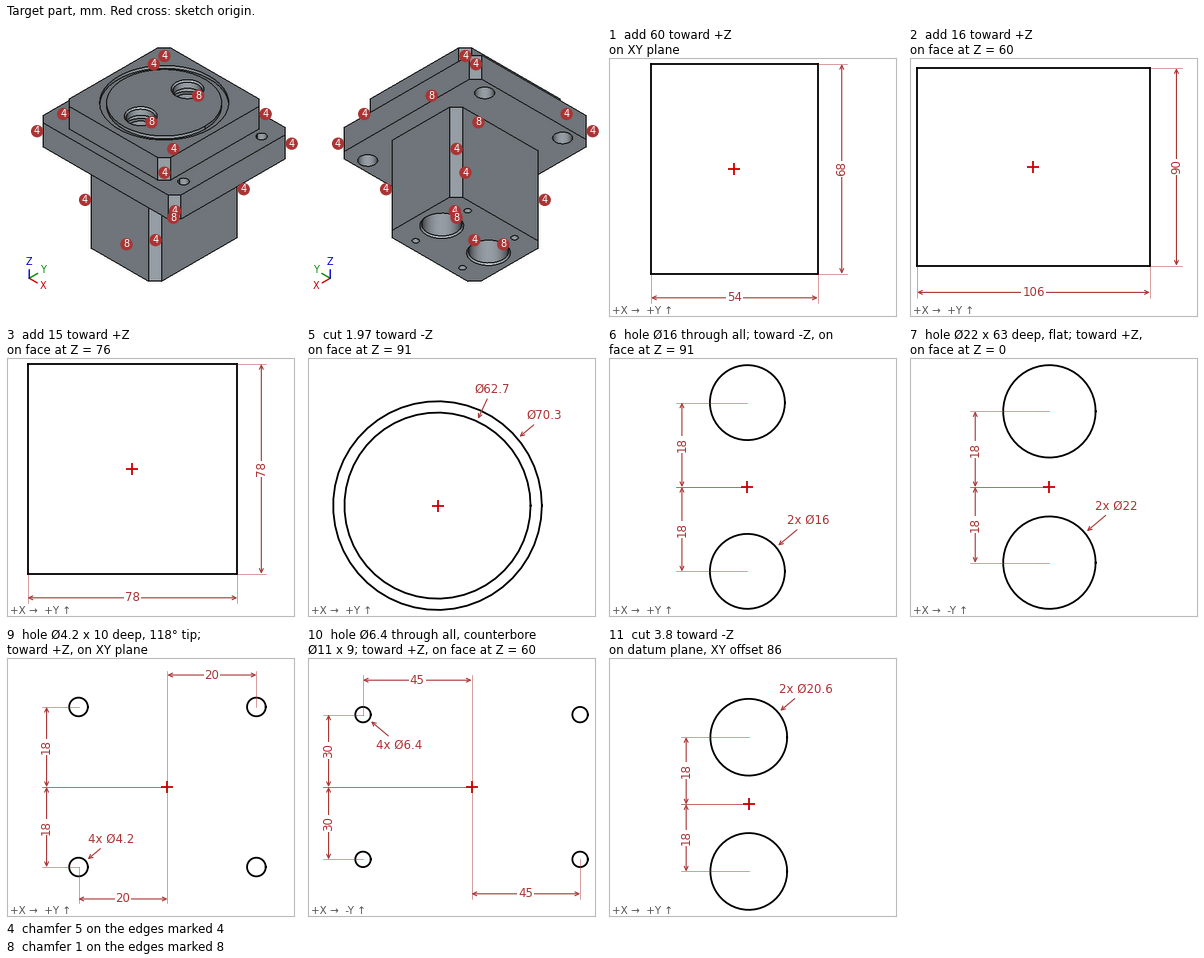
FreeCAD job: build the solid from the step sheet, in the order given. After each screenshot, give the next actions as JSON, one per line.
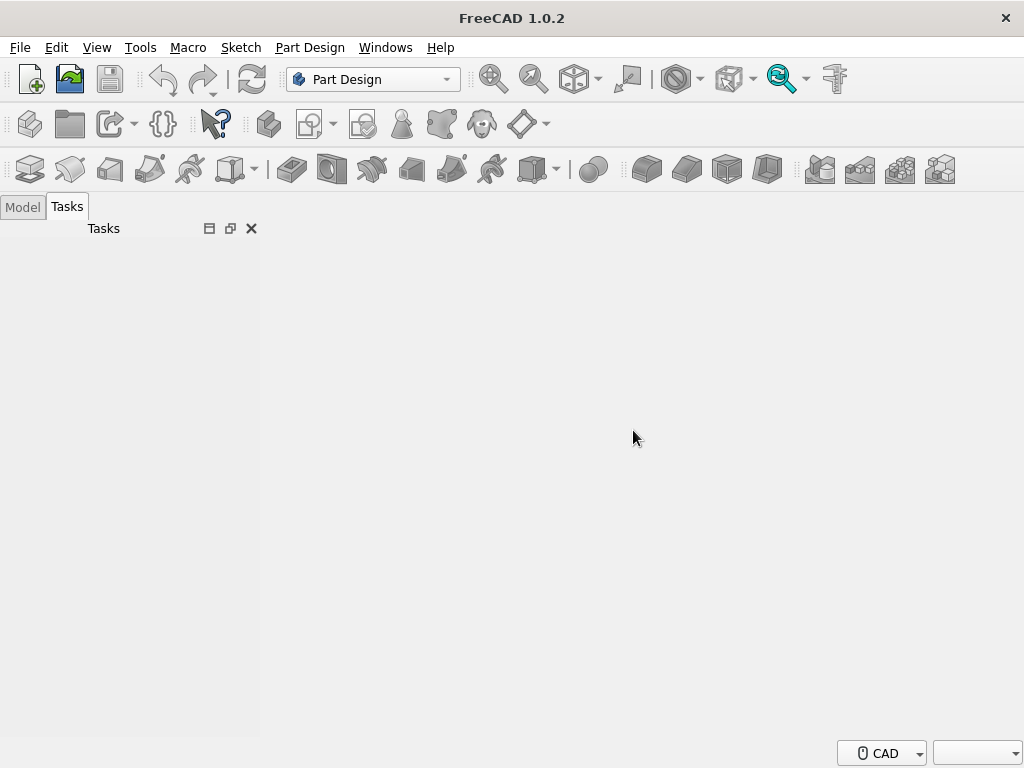
{"action": "key", "text": "ctrl+n"}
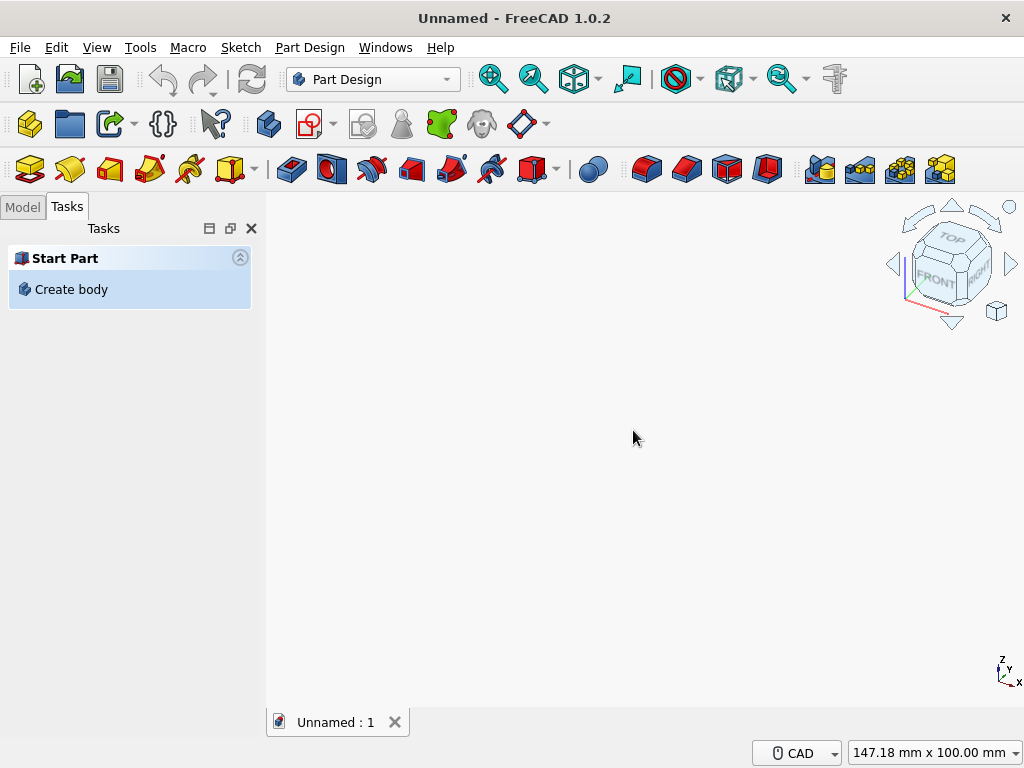
{"action": "left_click", "coordinate": [310, 124]}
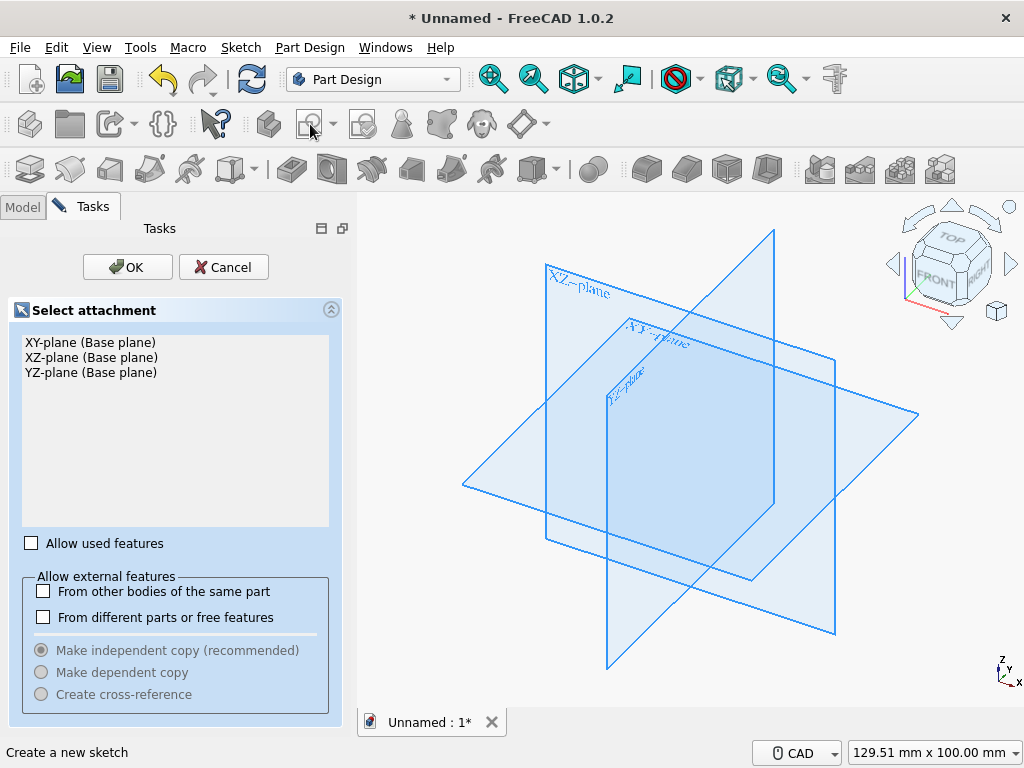
{"action": "left_click", "coordinate": [82, 342]}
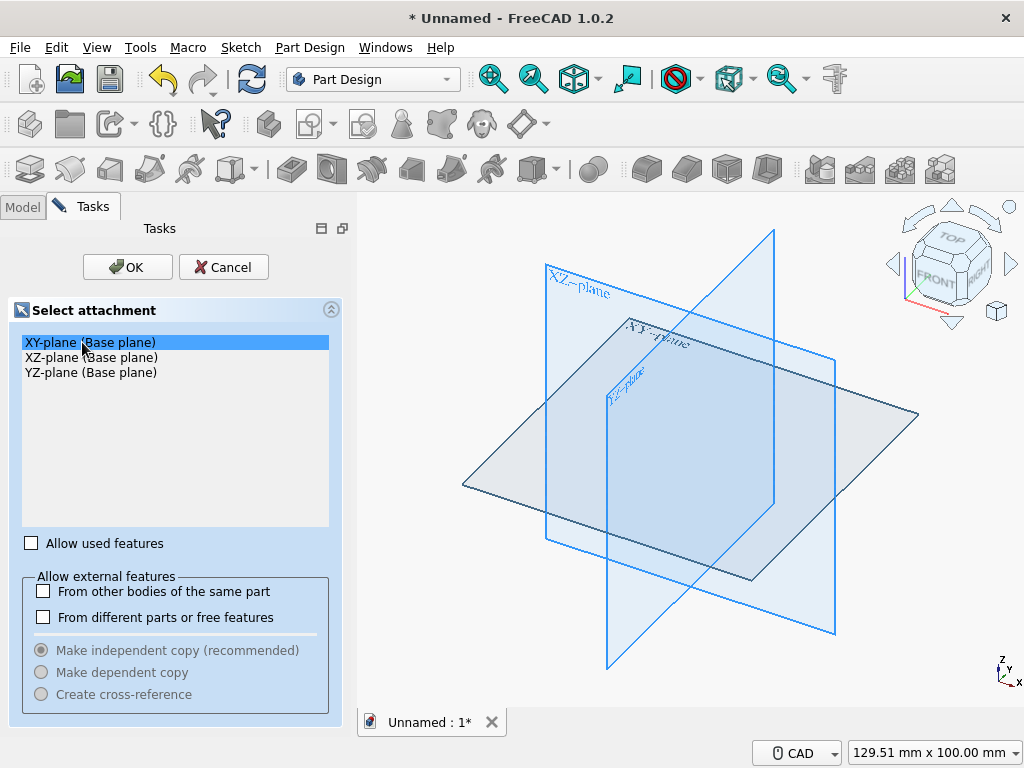
{"action": "left_click", "coordinate": [128, 267]}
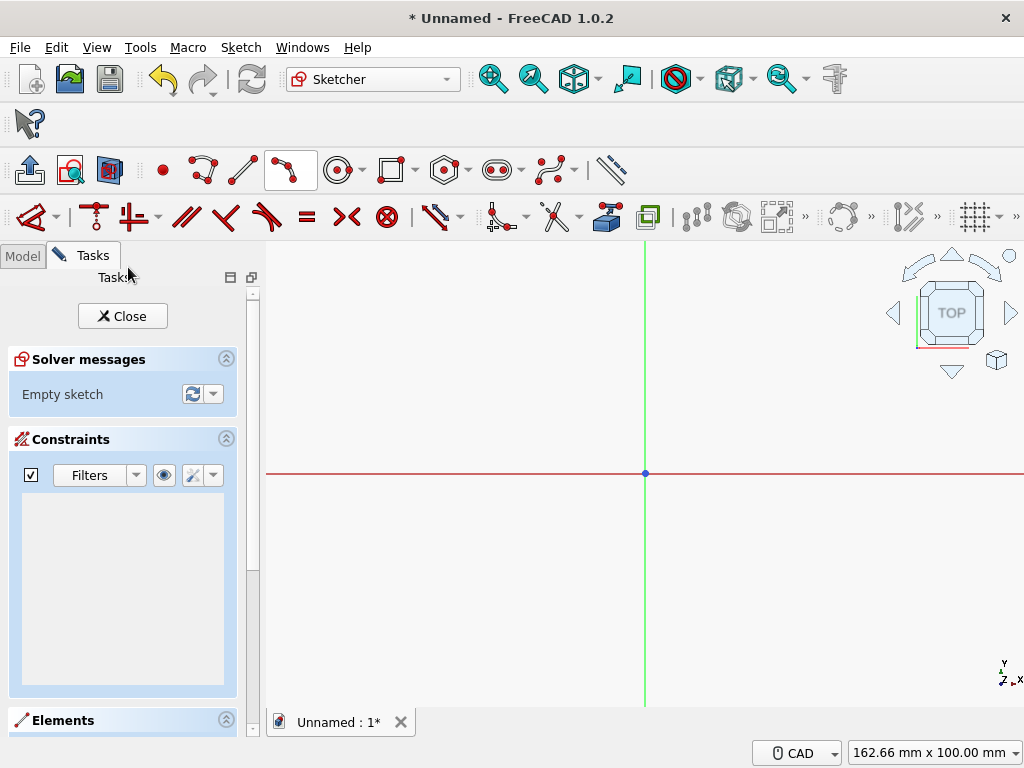
{"action": "key", "text": "g v"}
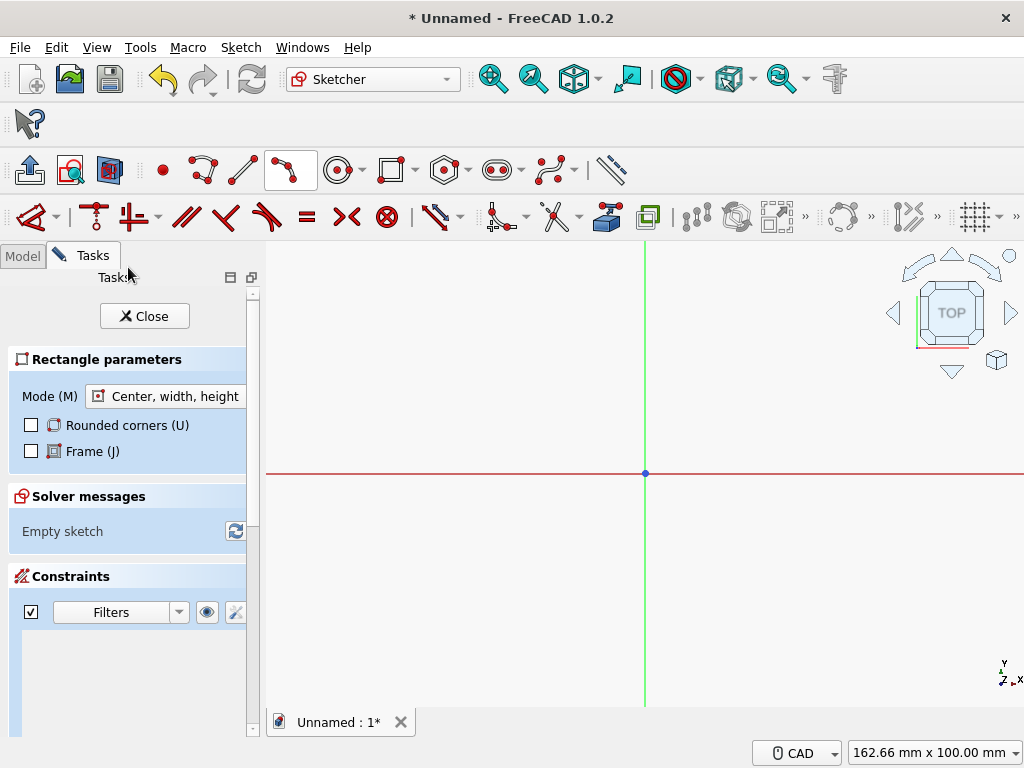
{"action": "left_click", "coordinate": [645, 474]}
{"action": "mouse_move", "coordinate": [771, 316]}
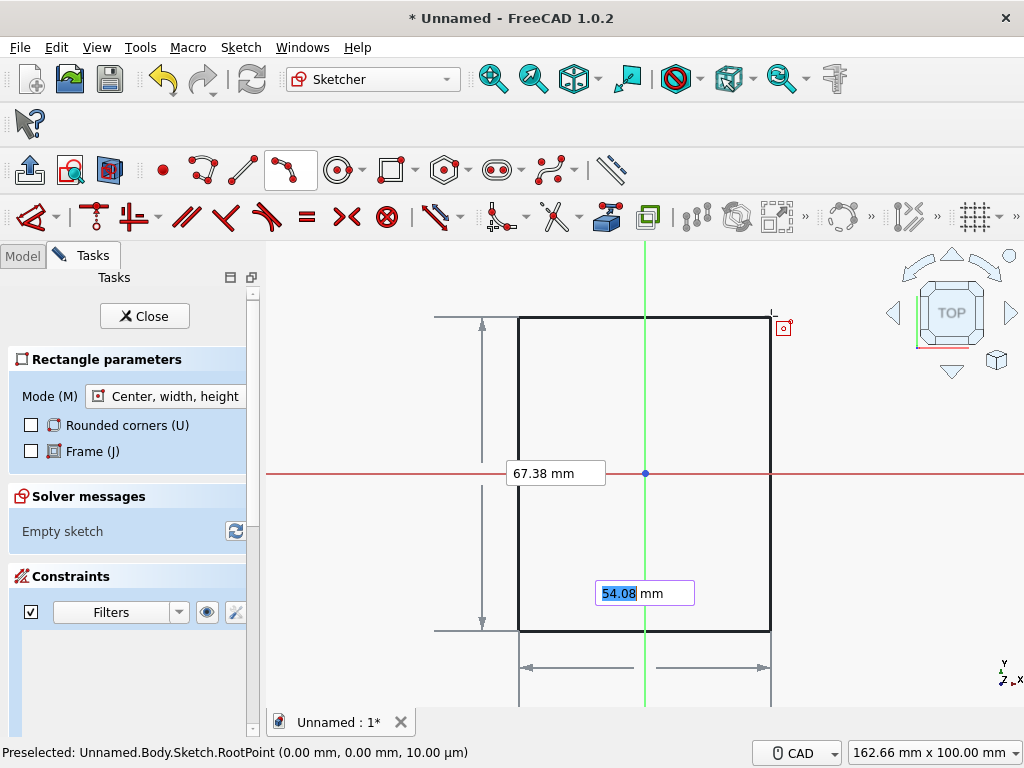
{"action": "type", "text": "54"}
{"action": "key", "text": "Tab"}
{"action": "type", "text": "68"}
{"action": "key", "text": "Return"}
{"action": "key", "text": "Escape"}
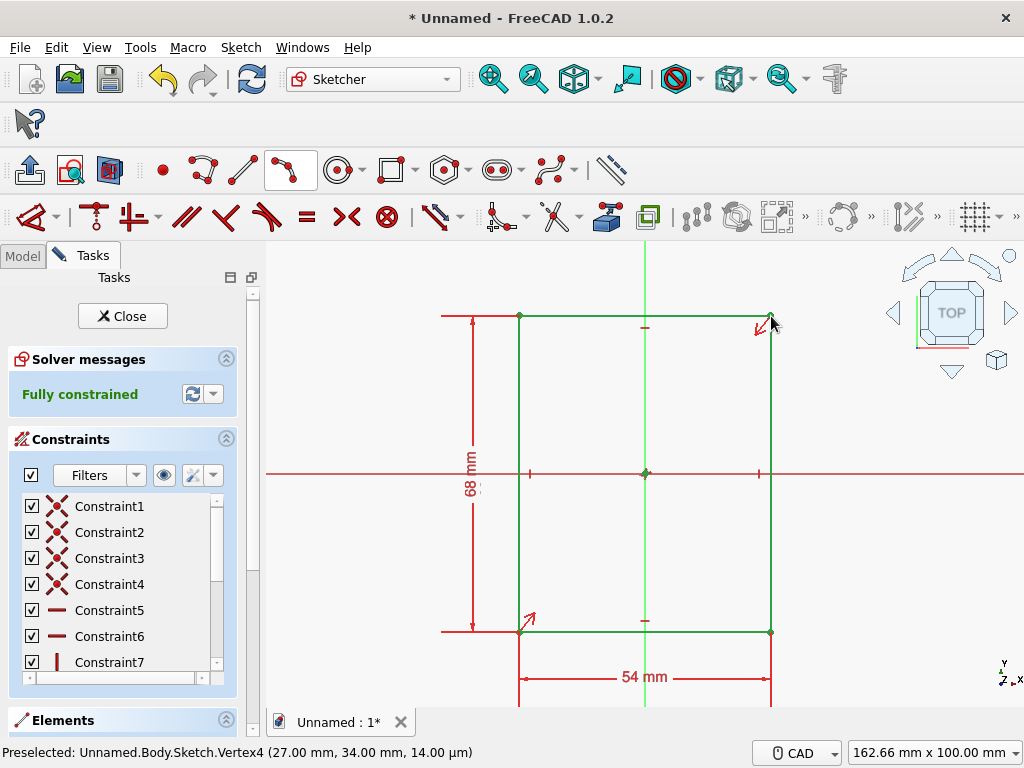
{"action": "left_click", "coordinate": [123, 316]}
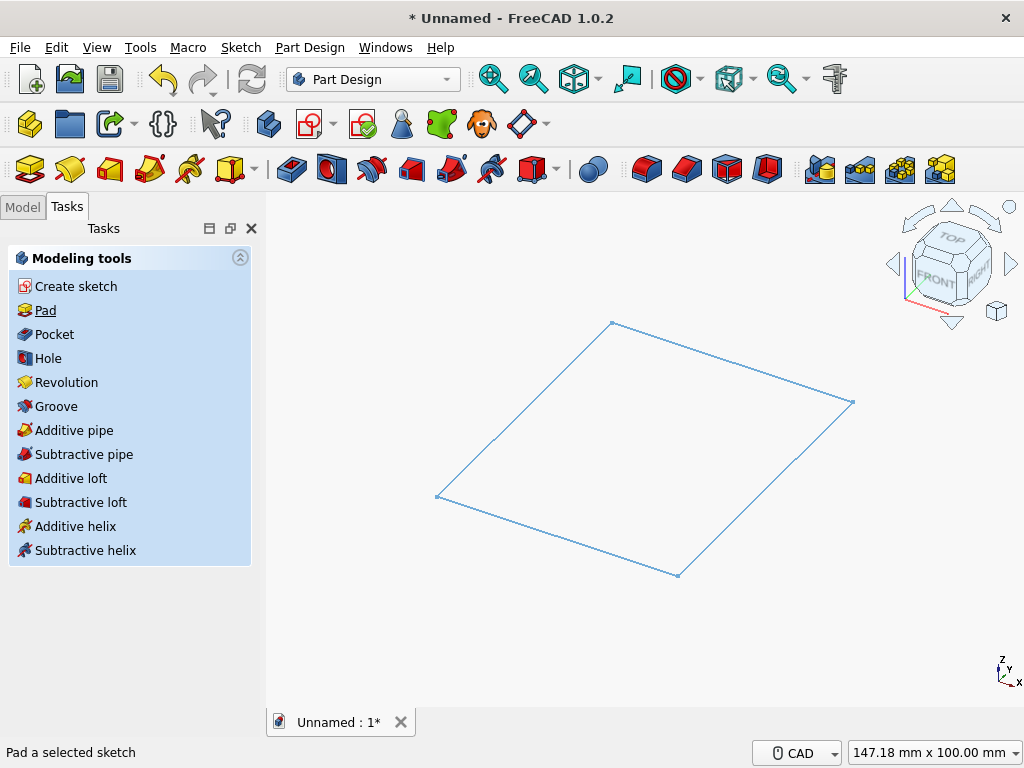
{"action": "left_click", "coordinate": [30, 170]}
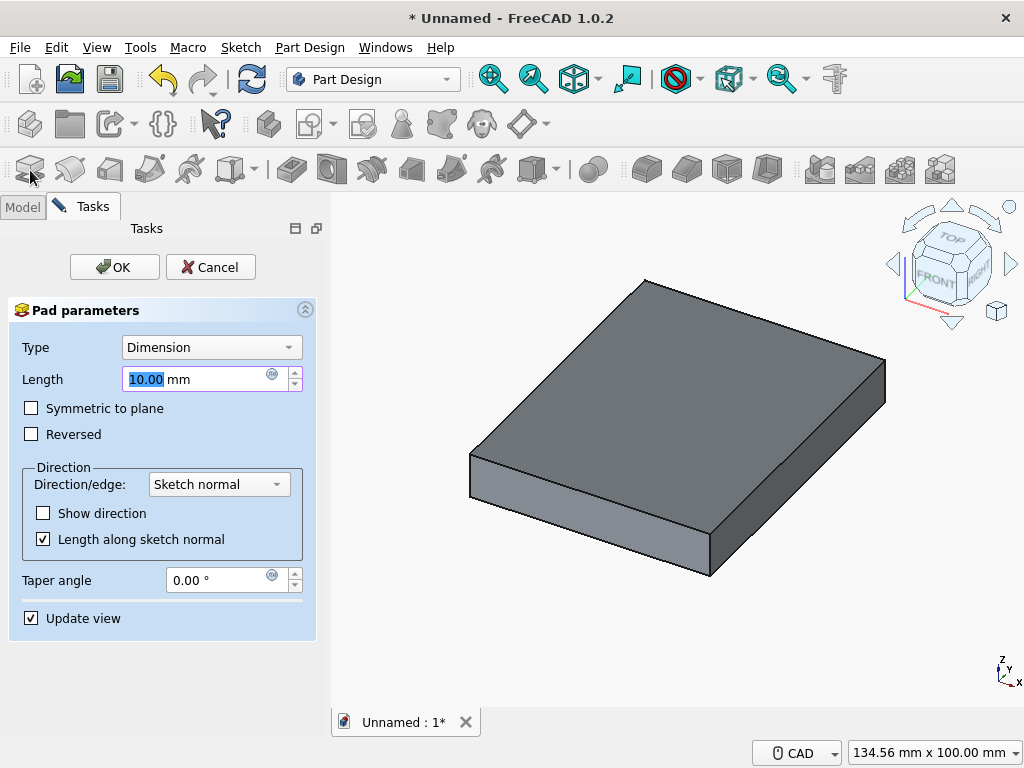
{"action": "type", "text": "60"}
{"action": "key", "text": "Tab"}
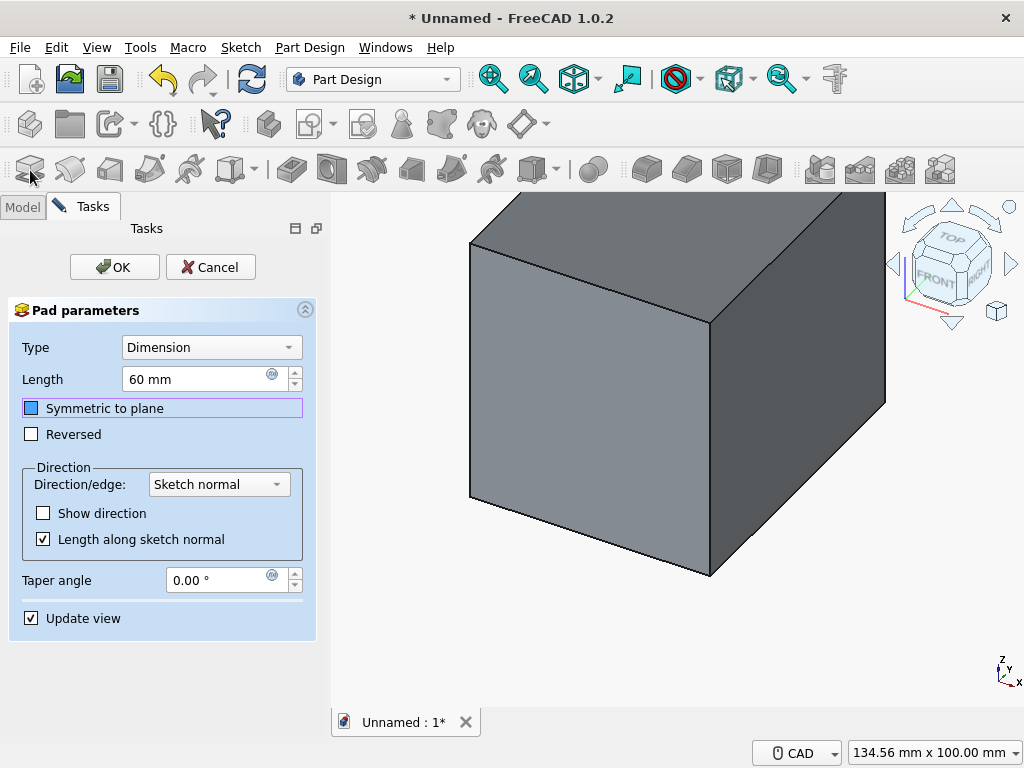
{"action": "left_click", "coordinate": [115, 267]}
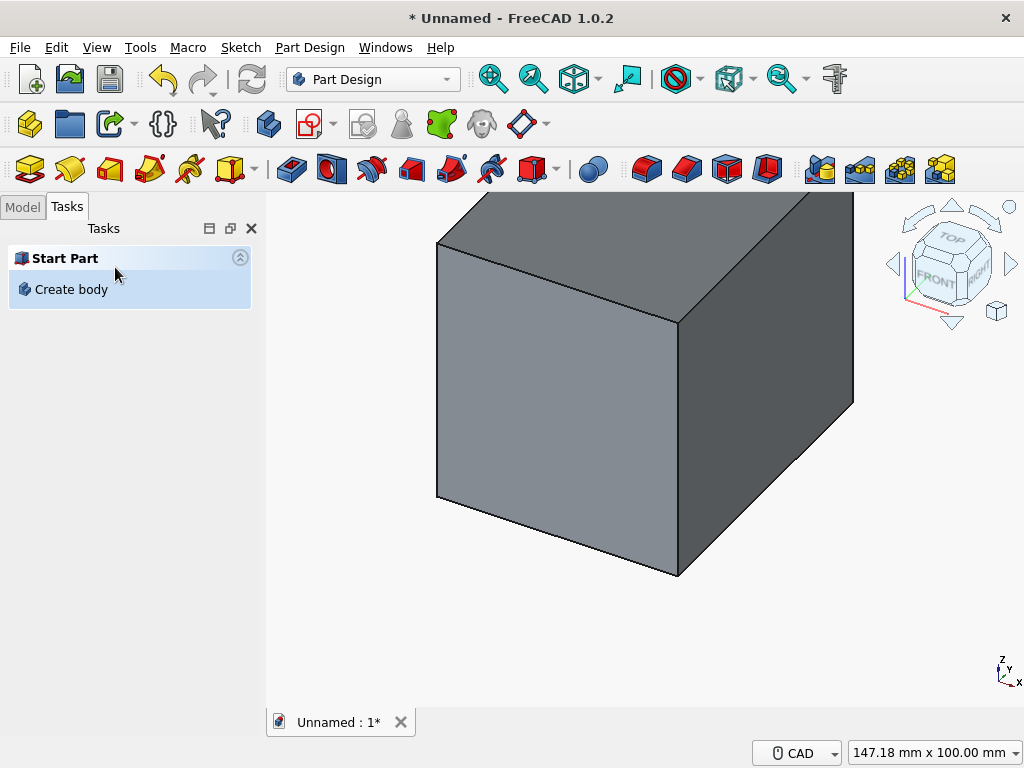
{"action": "key", "text": "v f"}